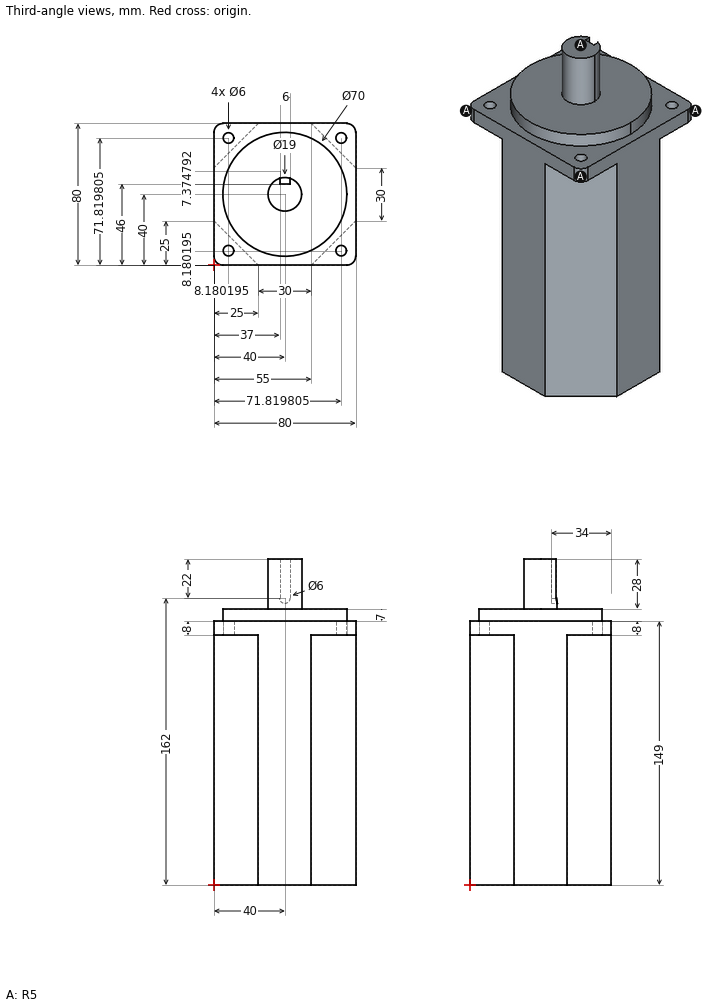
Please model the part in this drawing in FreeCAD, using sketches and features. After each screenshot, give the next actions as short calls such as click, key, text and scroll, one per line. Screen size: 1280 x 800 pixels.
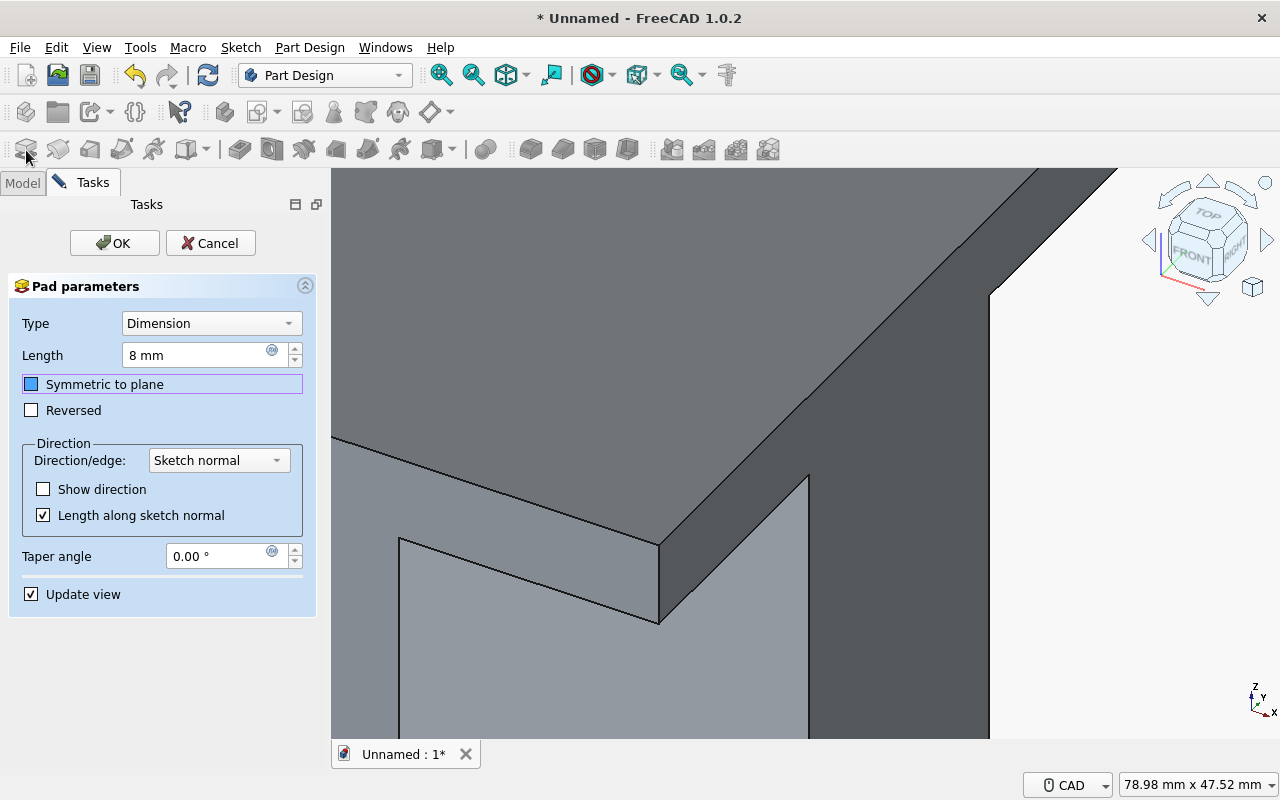
click(30, 410)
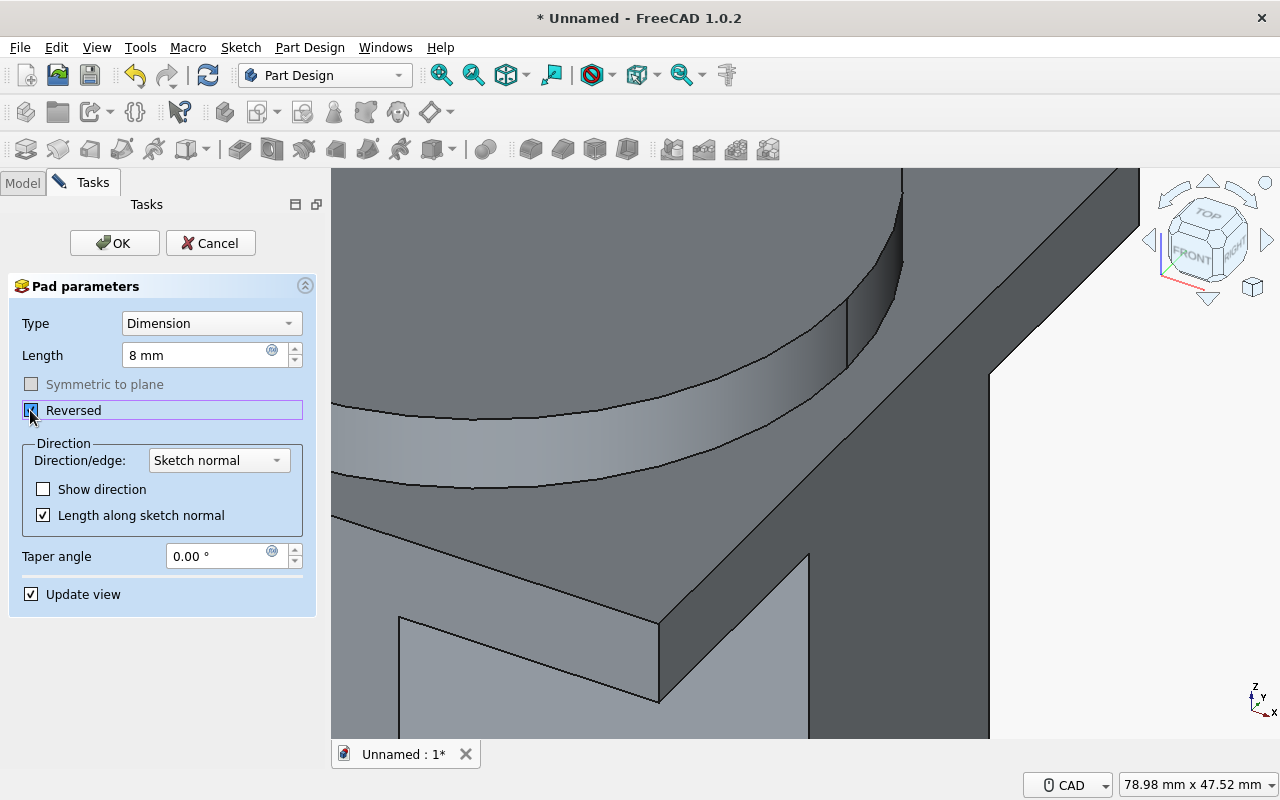
click(115, 243)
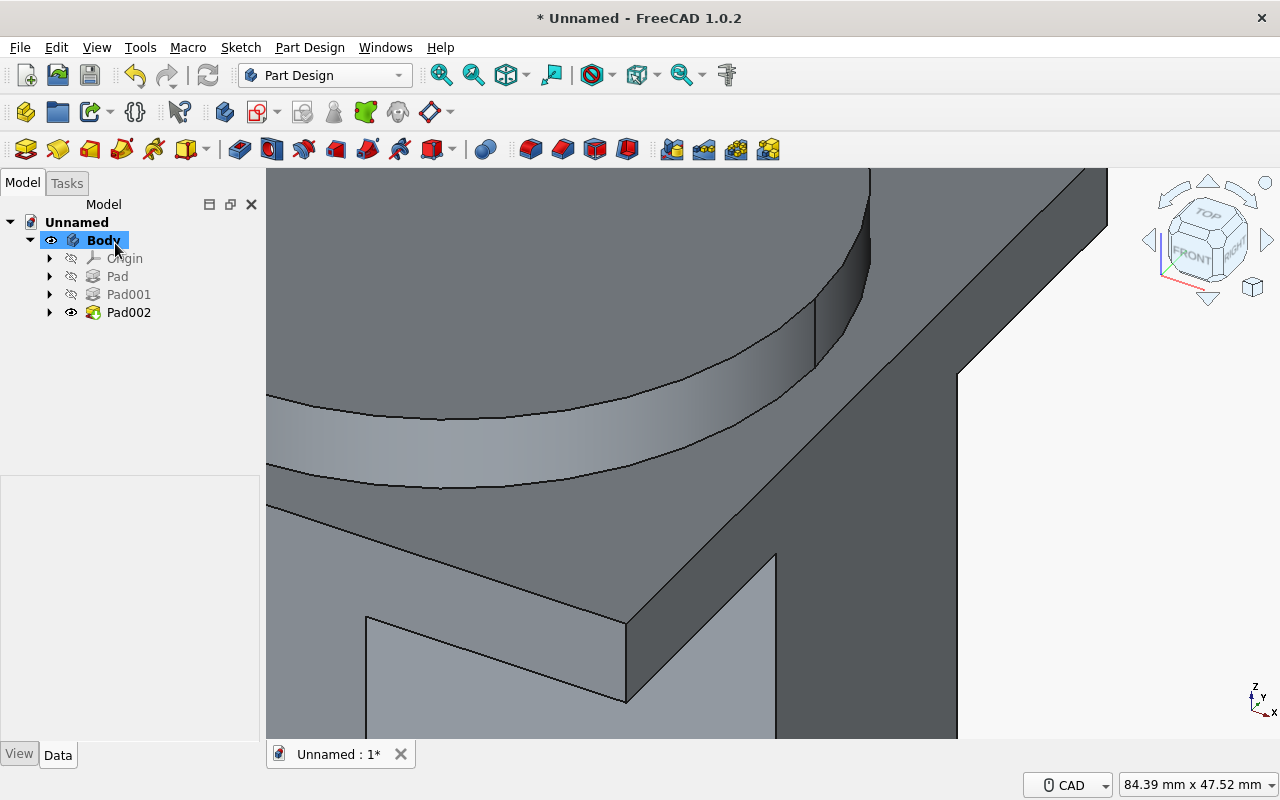
click(442, 76)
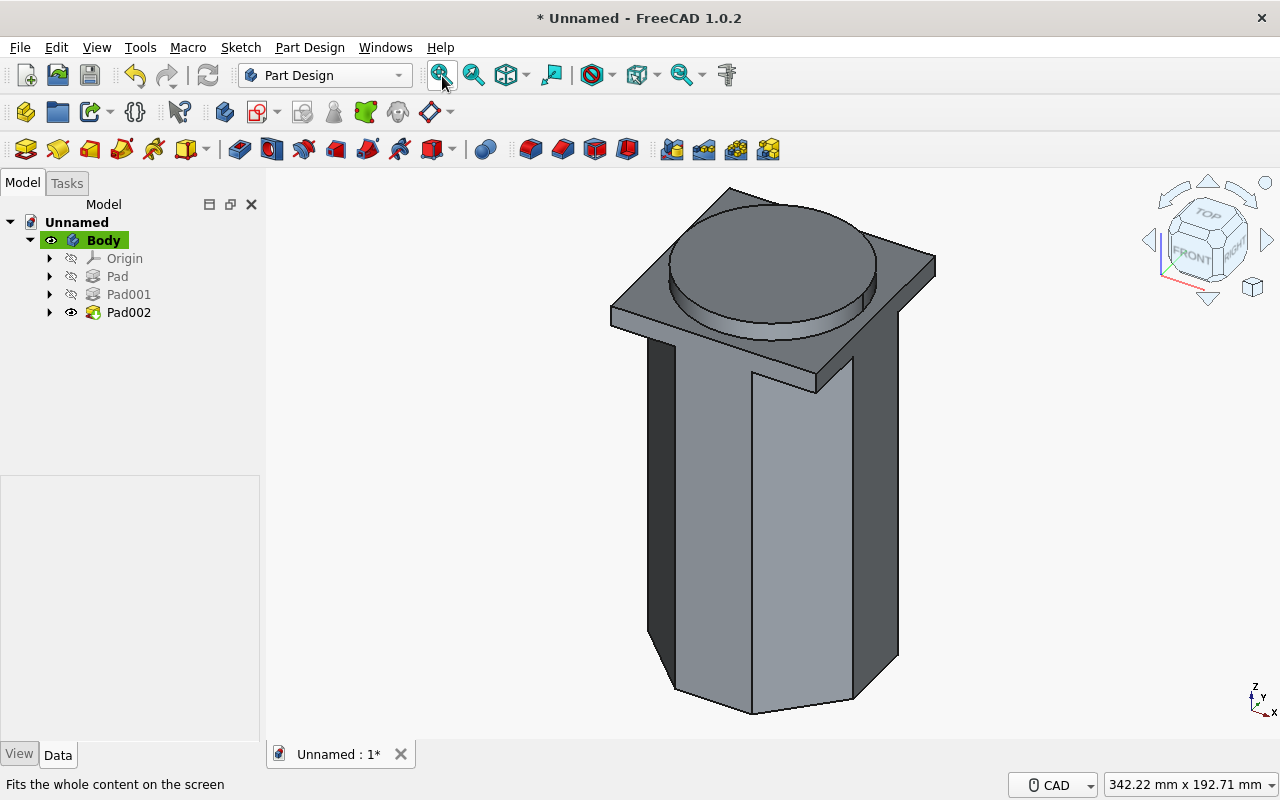
click(781, 350)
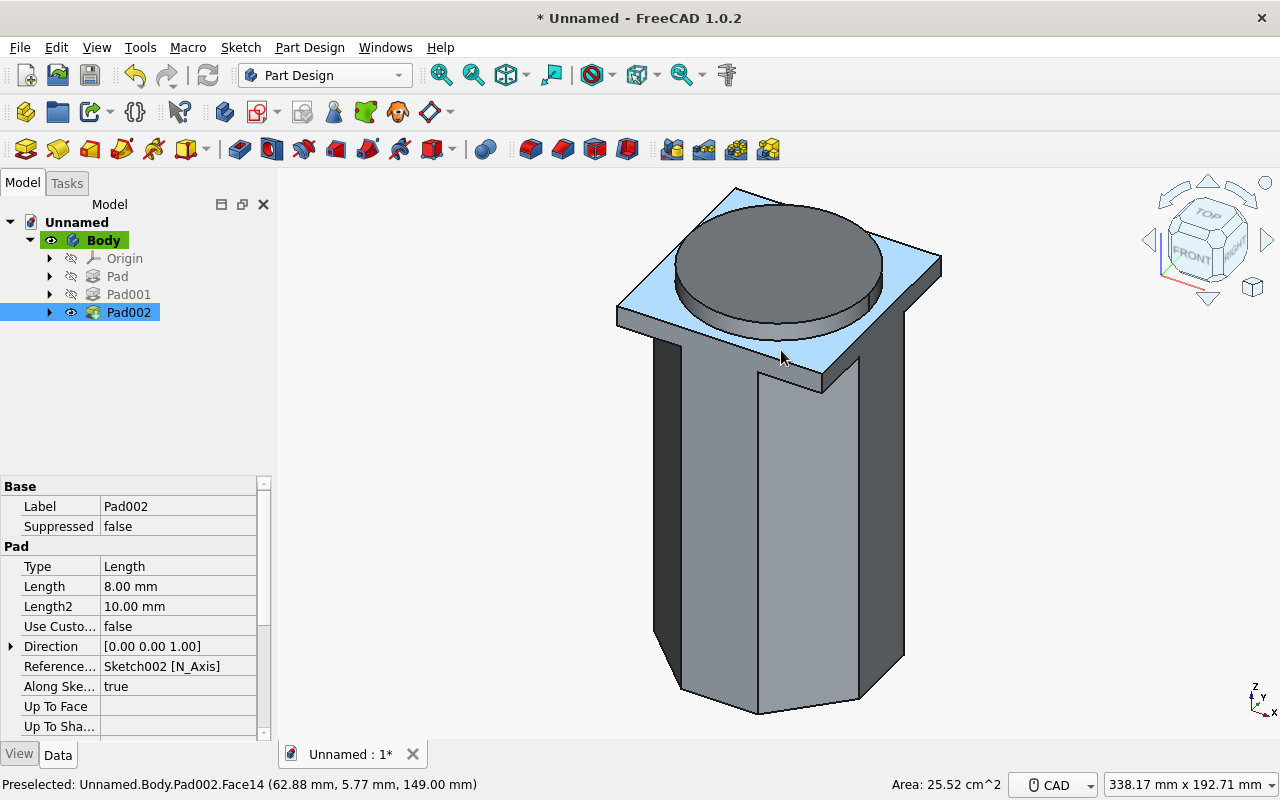
click(258, 112)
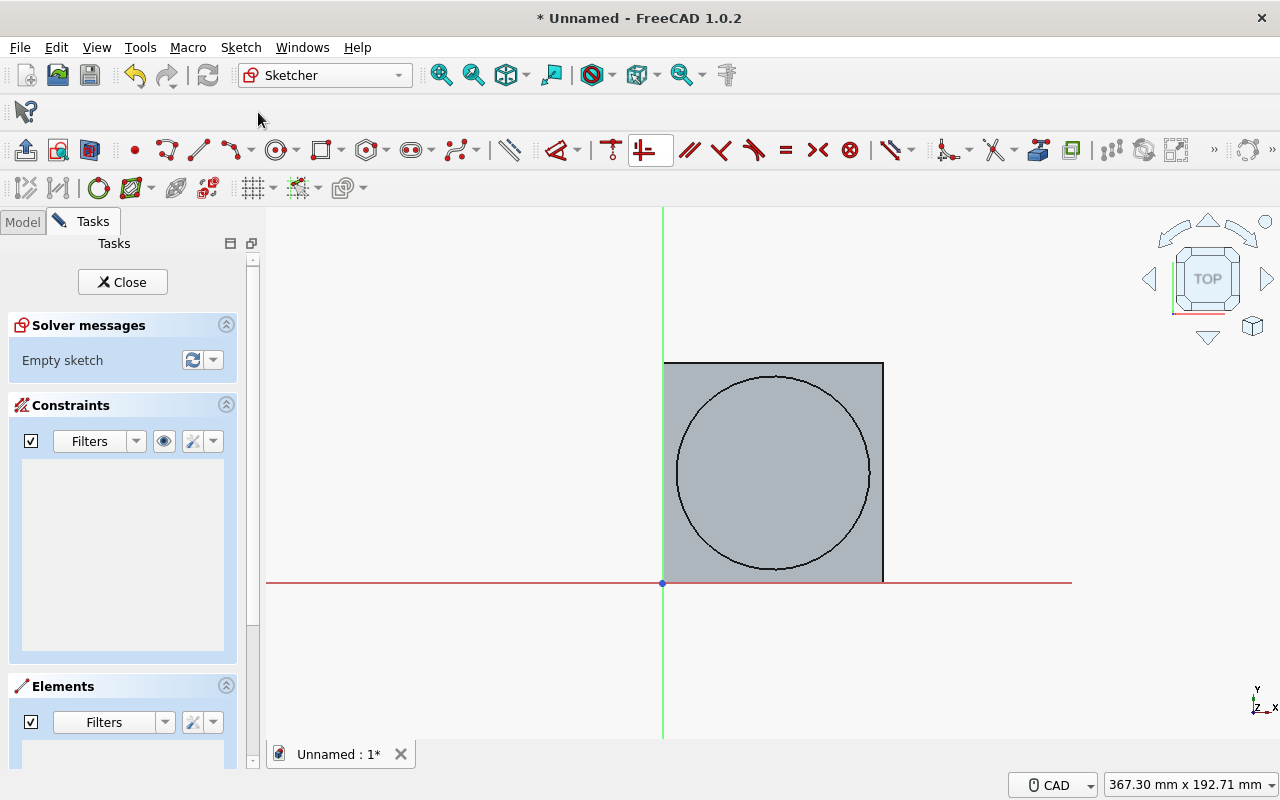
scroll(891, 495, up, 2)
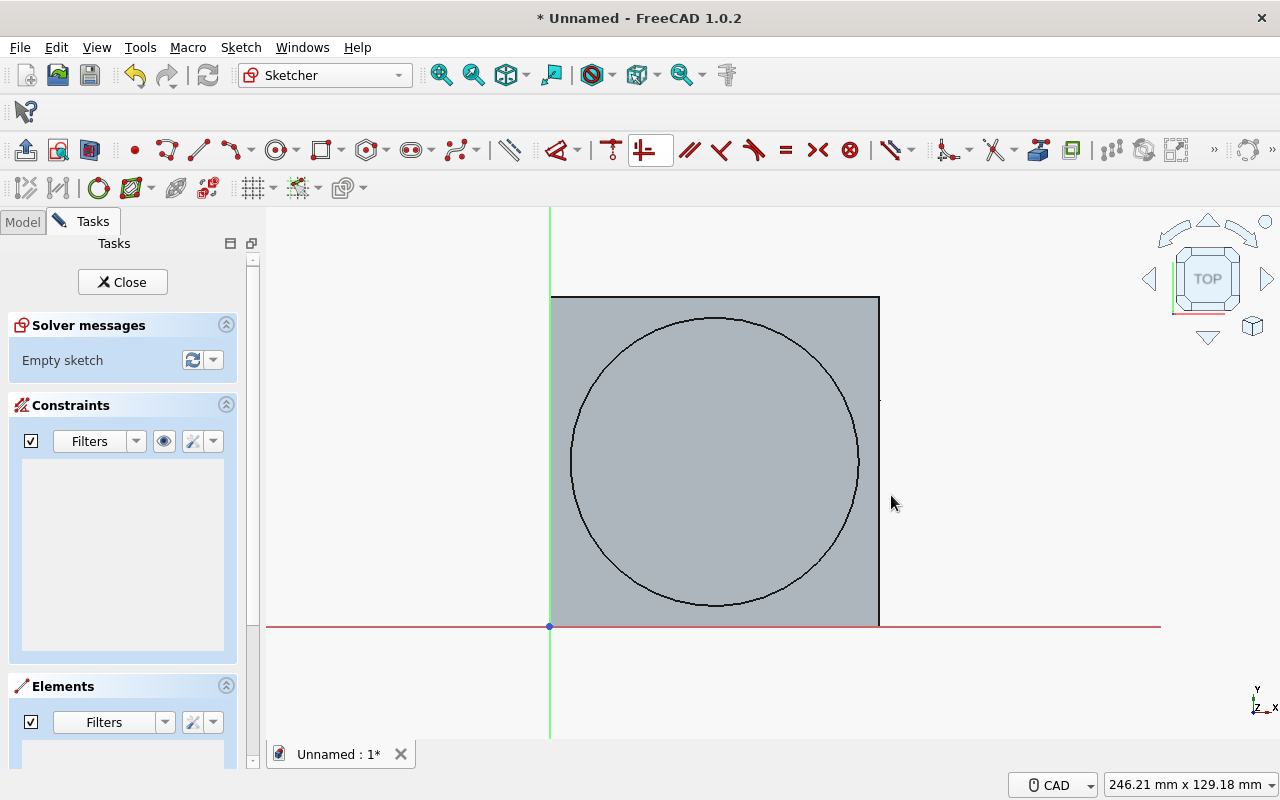
key(g)
key(c)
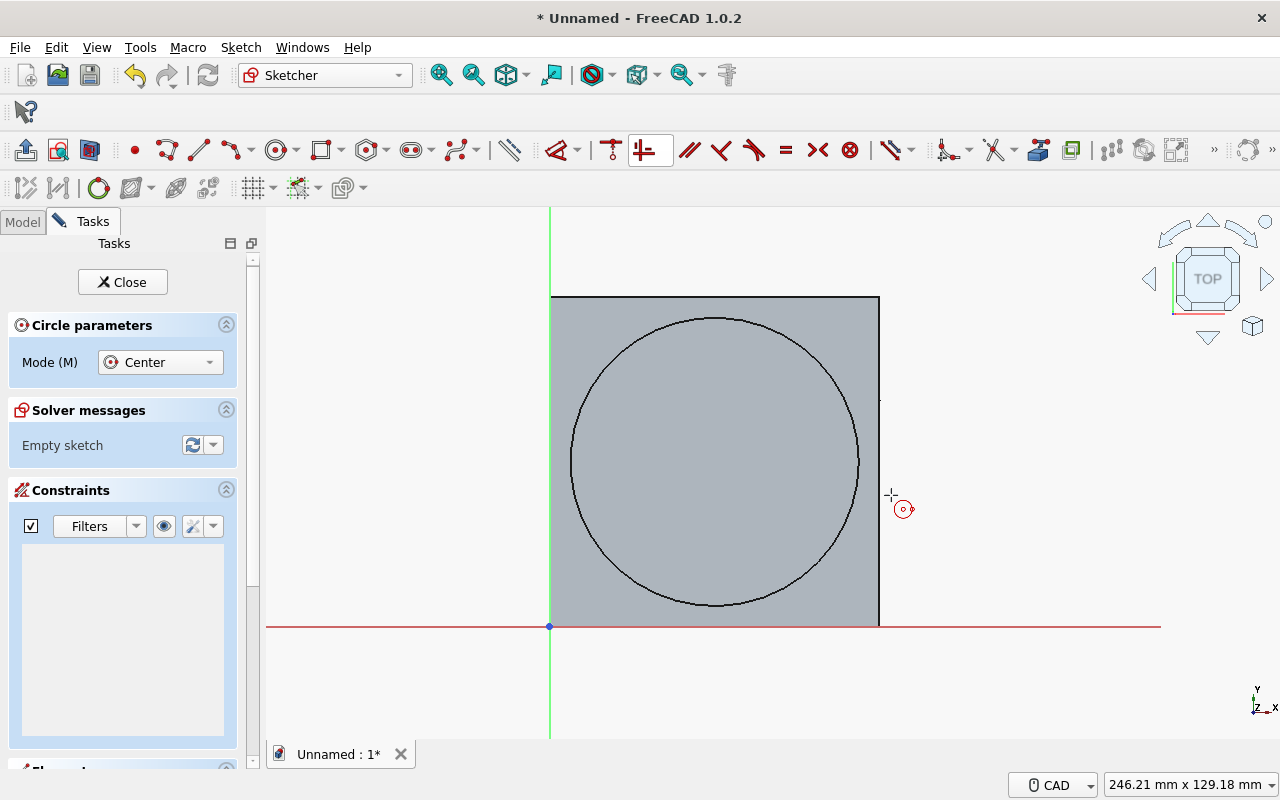
scroll(584, 331, up, 4)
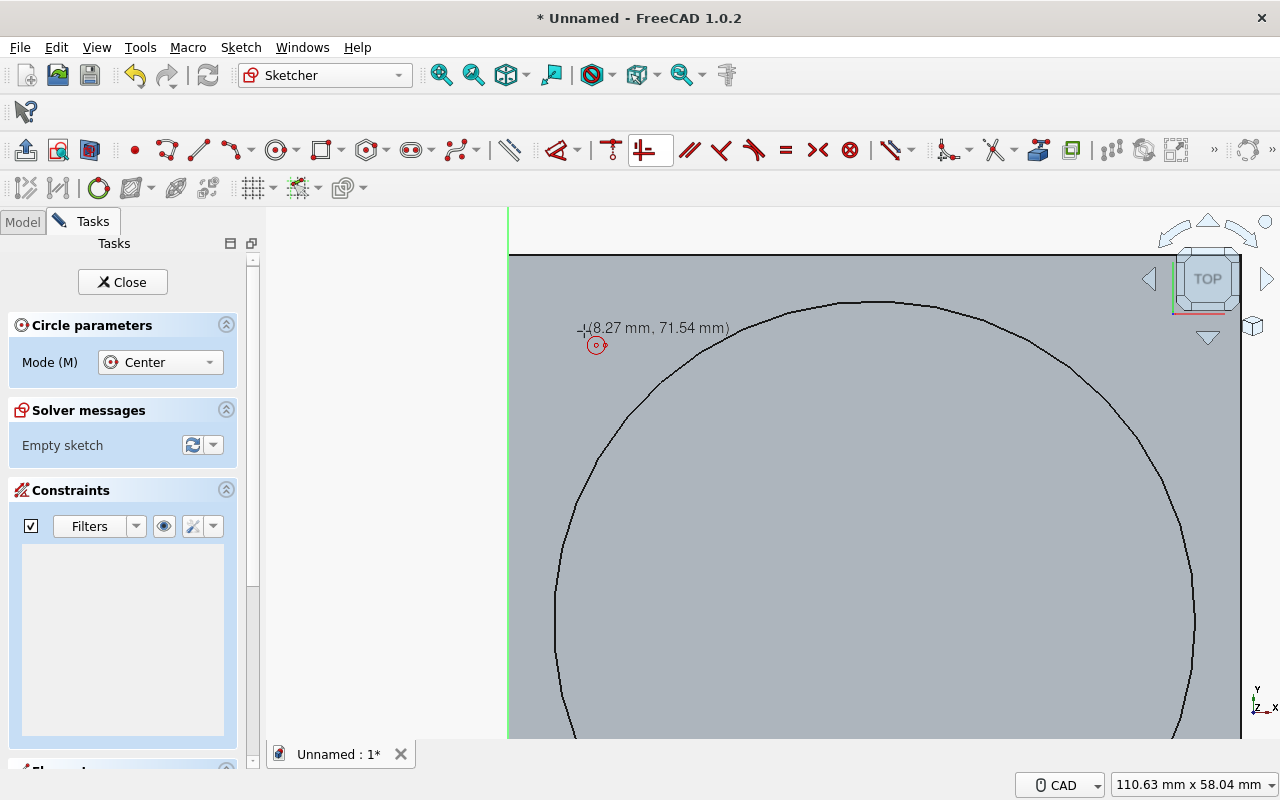
click(583, 330)
click(602, 311)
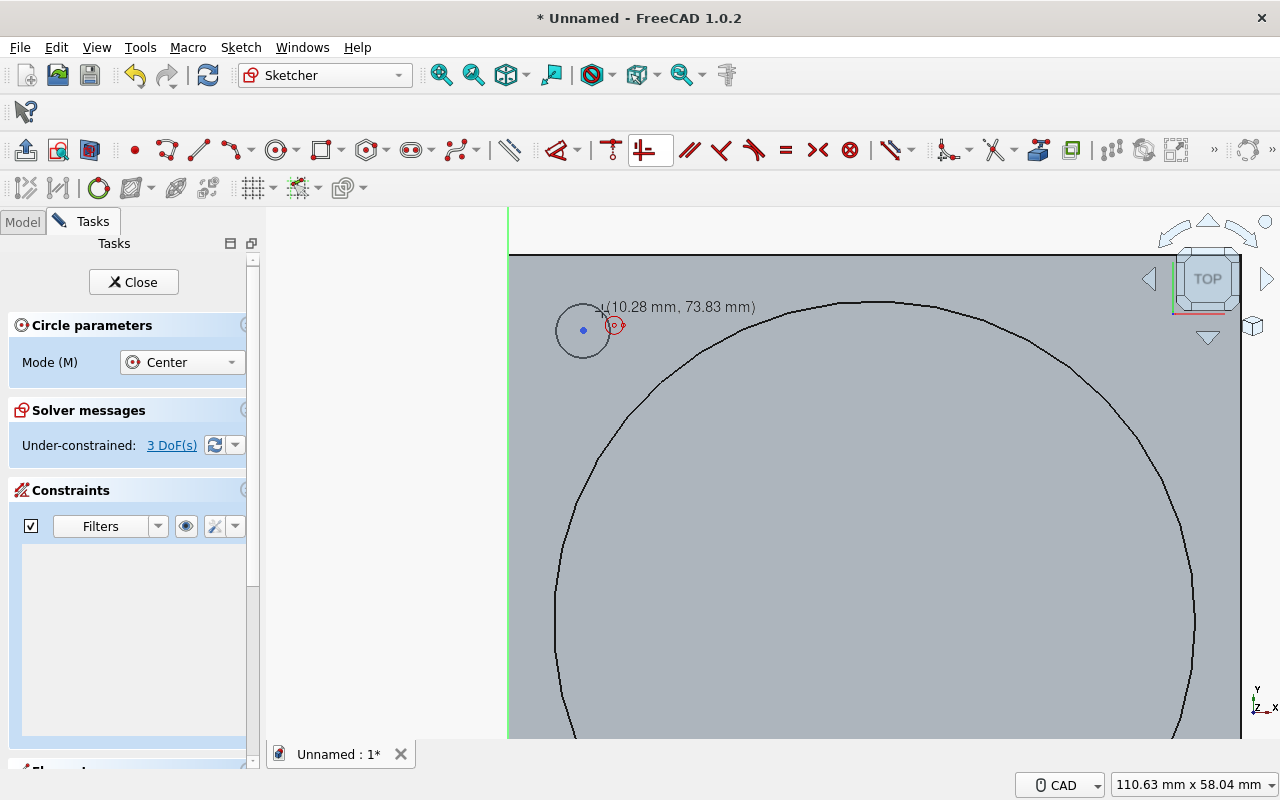
scroll(585, 332, down, 4)